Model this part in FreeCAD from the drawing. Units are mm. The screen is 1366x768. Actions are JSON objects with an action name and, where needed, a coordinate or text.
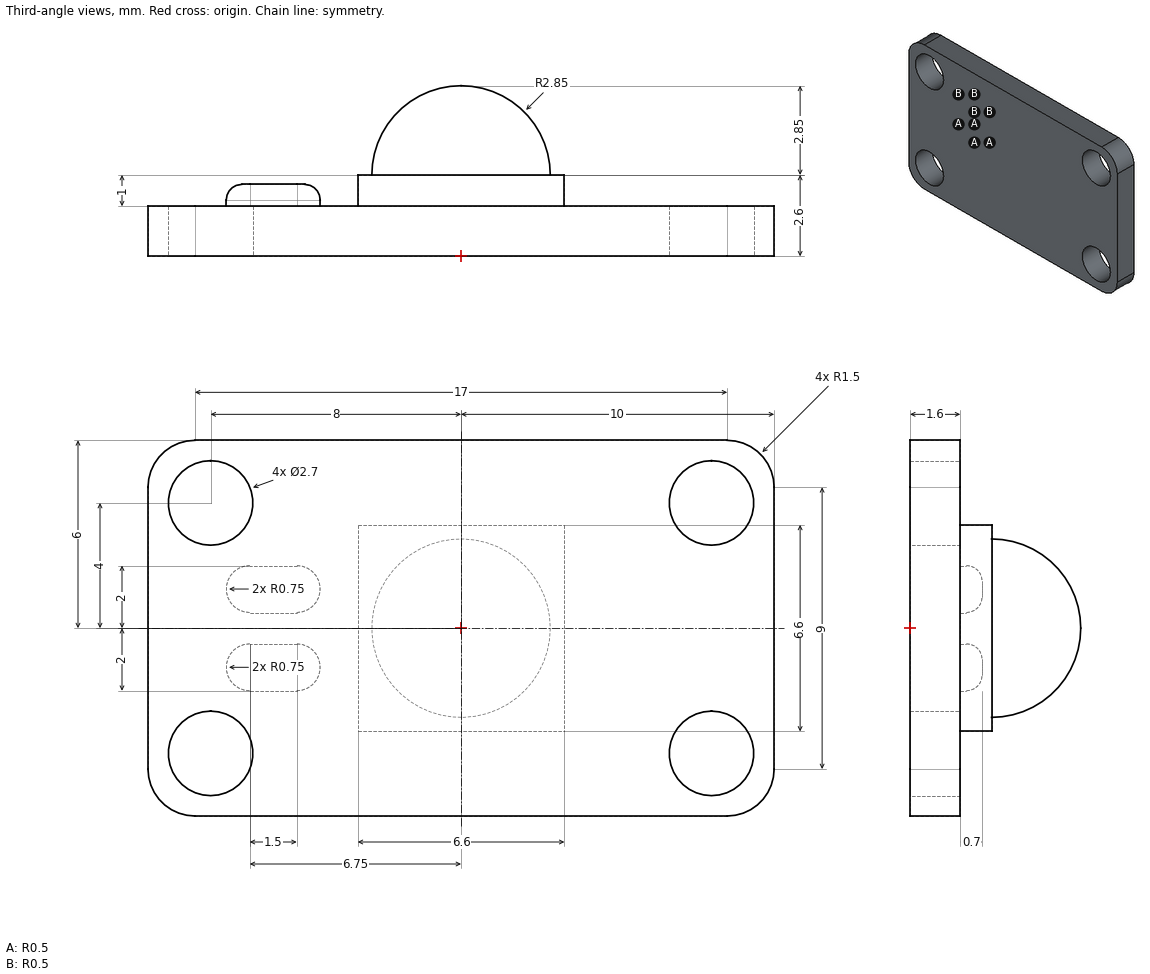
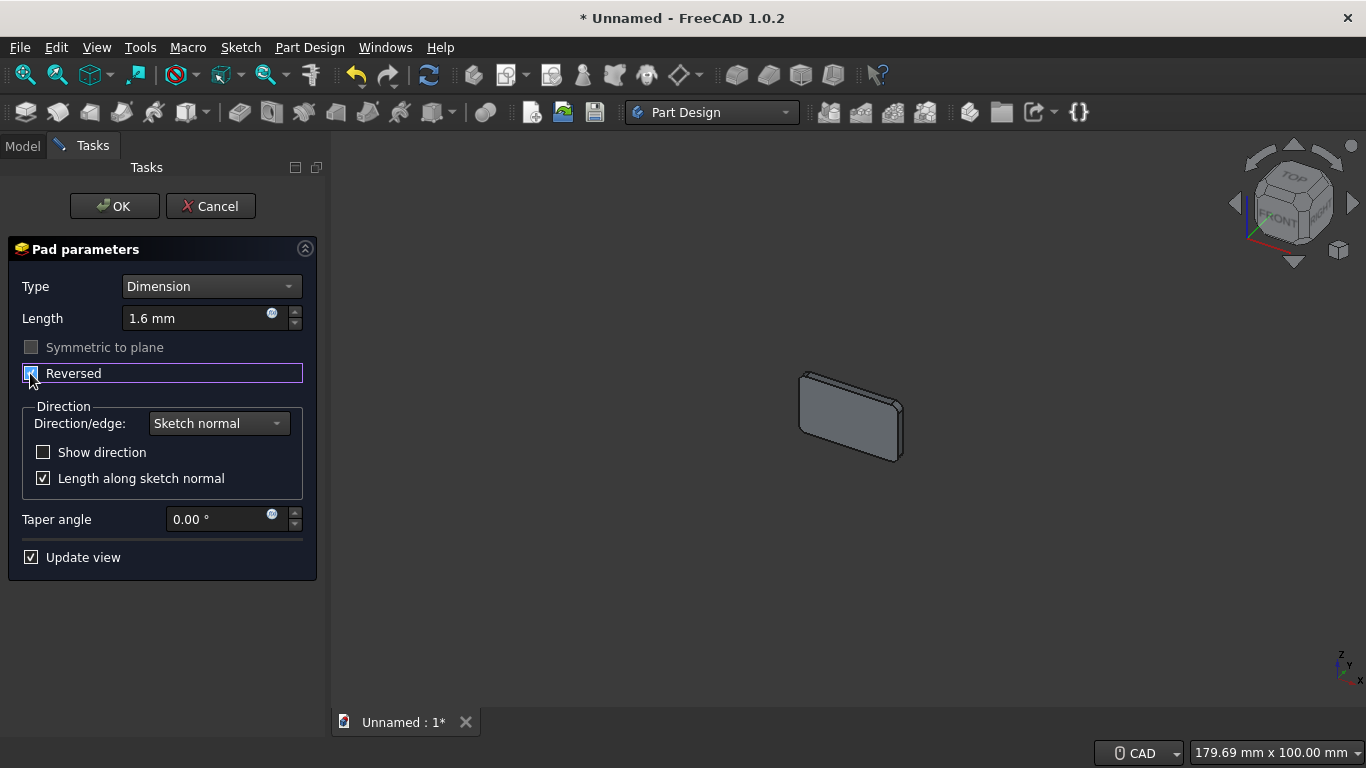
{"action": "left_click", "coordinate": [115, 206]}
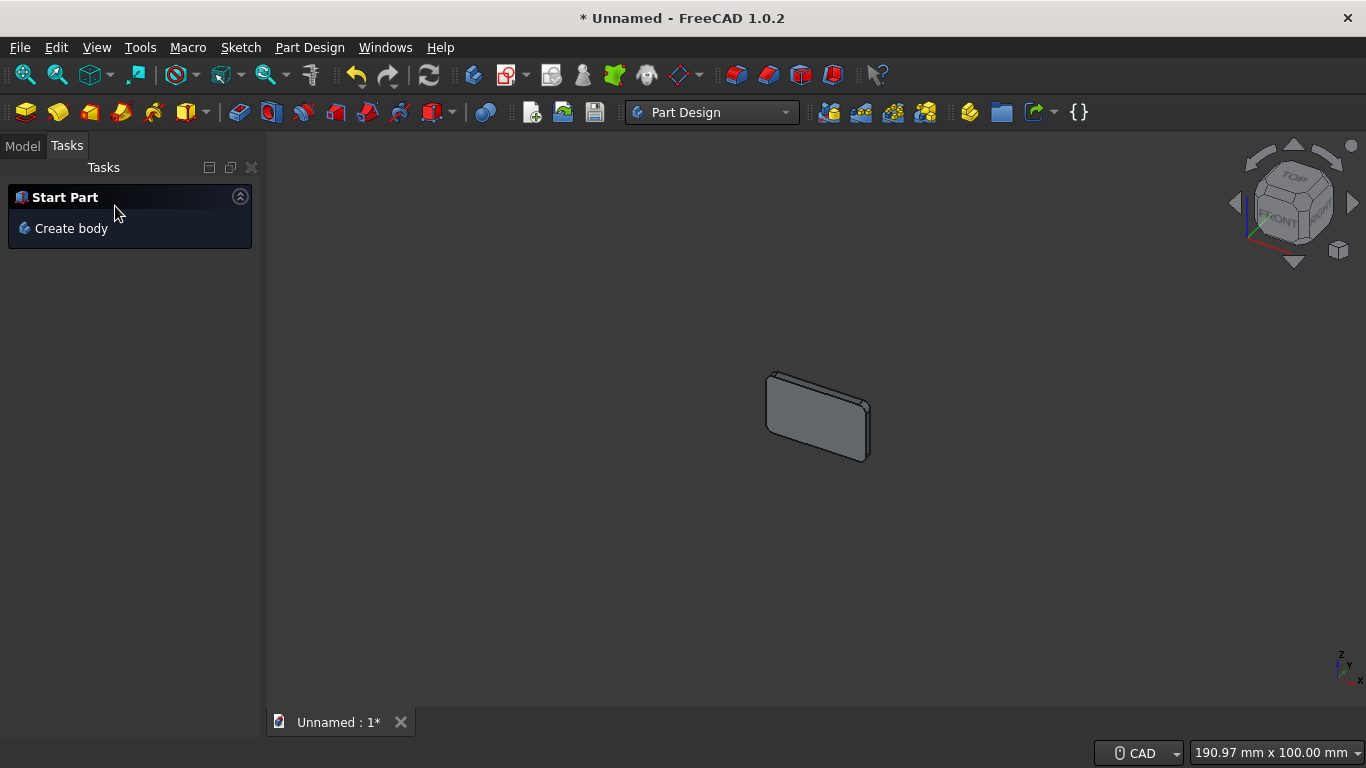
{"action": "key", "text": "v f"}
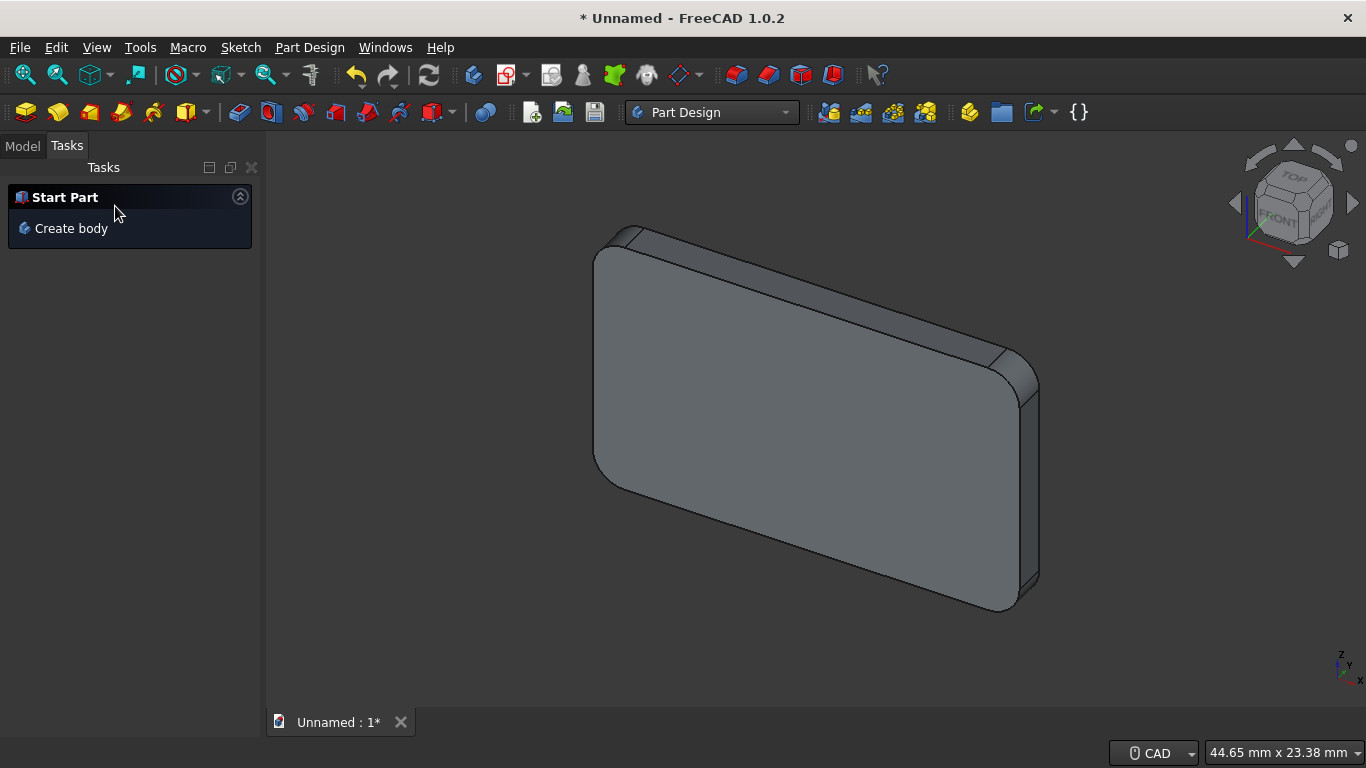
{"action": "left_click", "coordinate": [506, 76]}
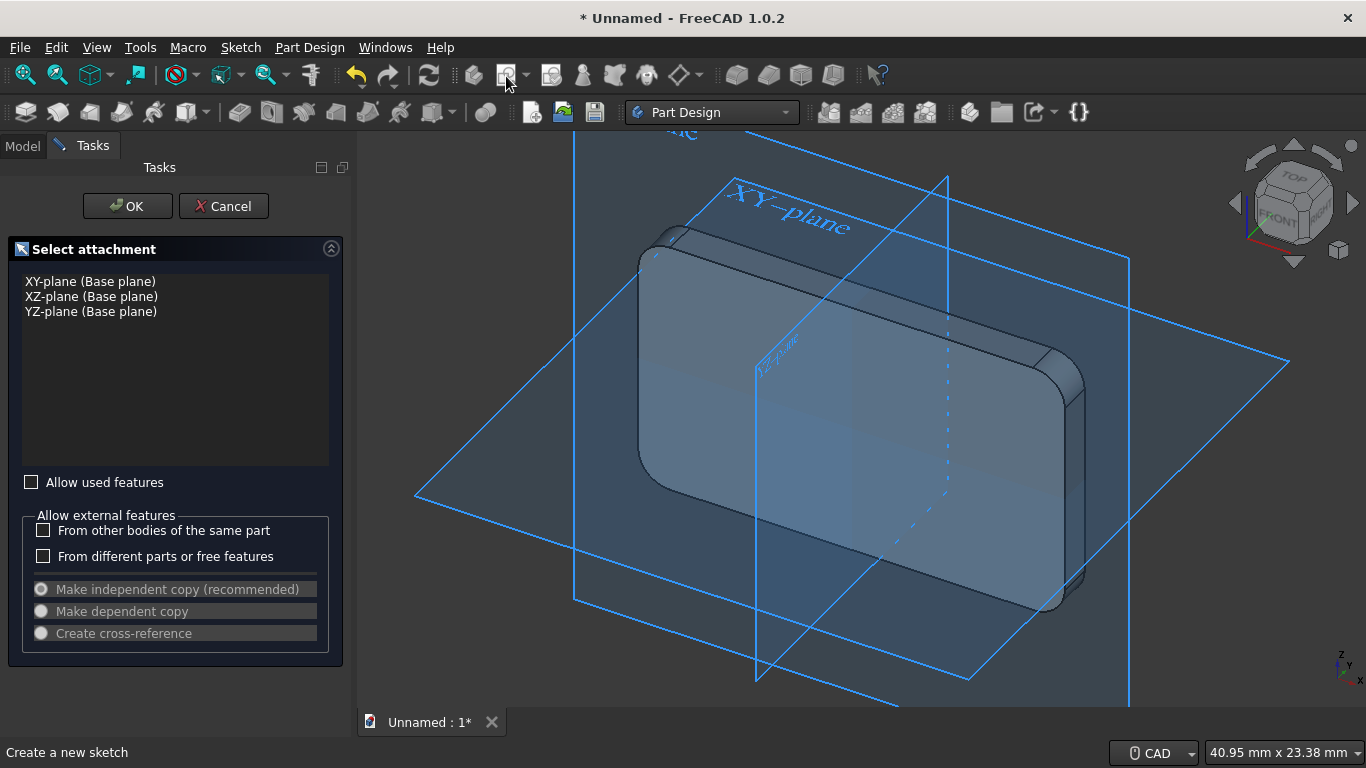
{"action": "left_click", "coordinate": [82, 296]}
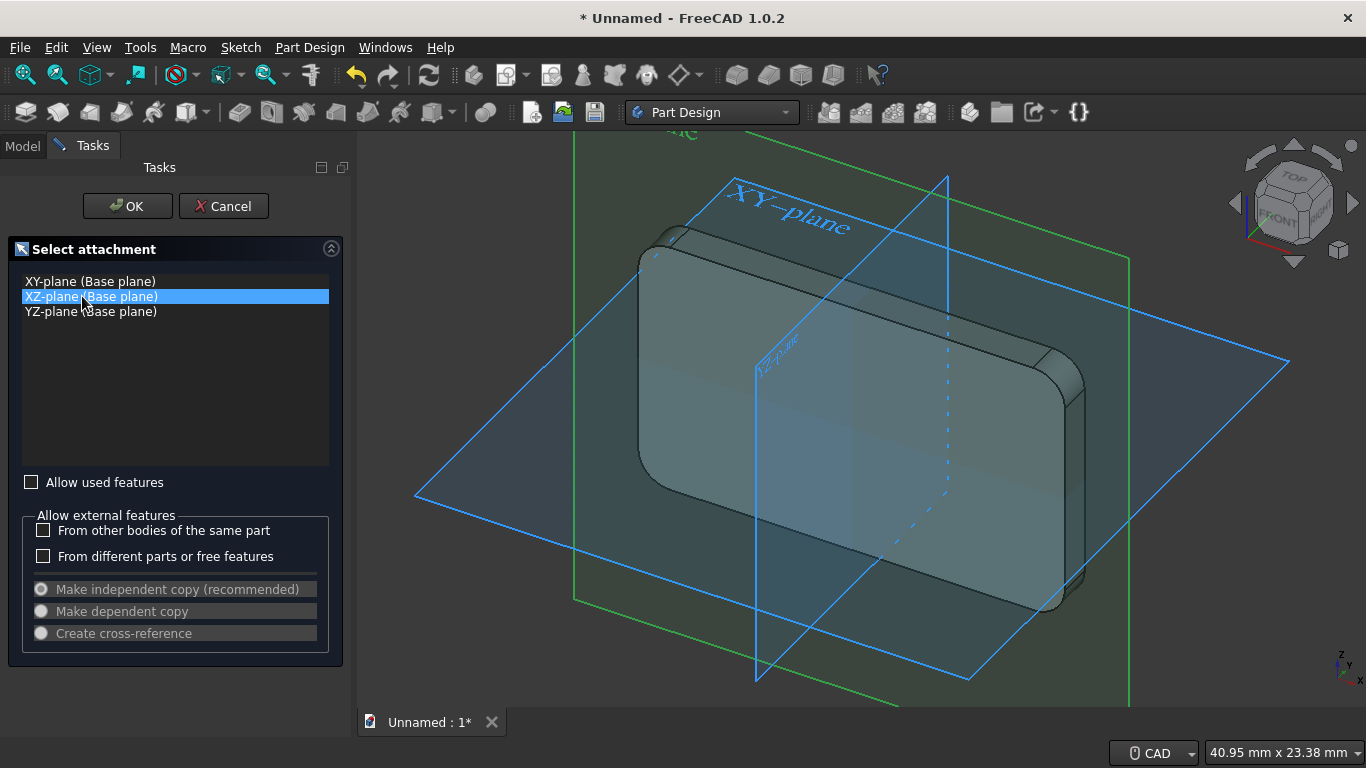
{"action": "left_click", "coordinate": [128, 206]}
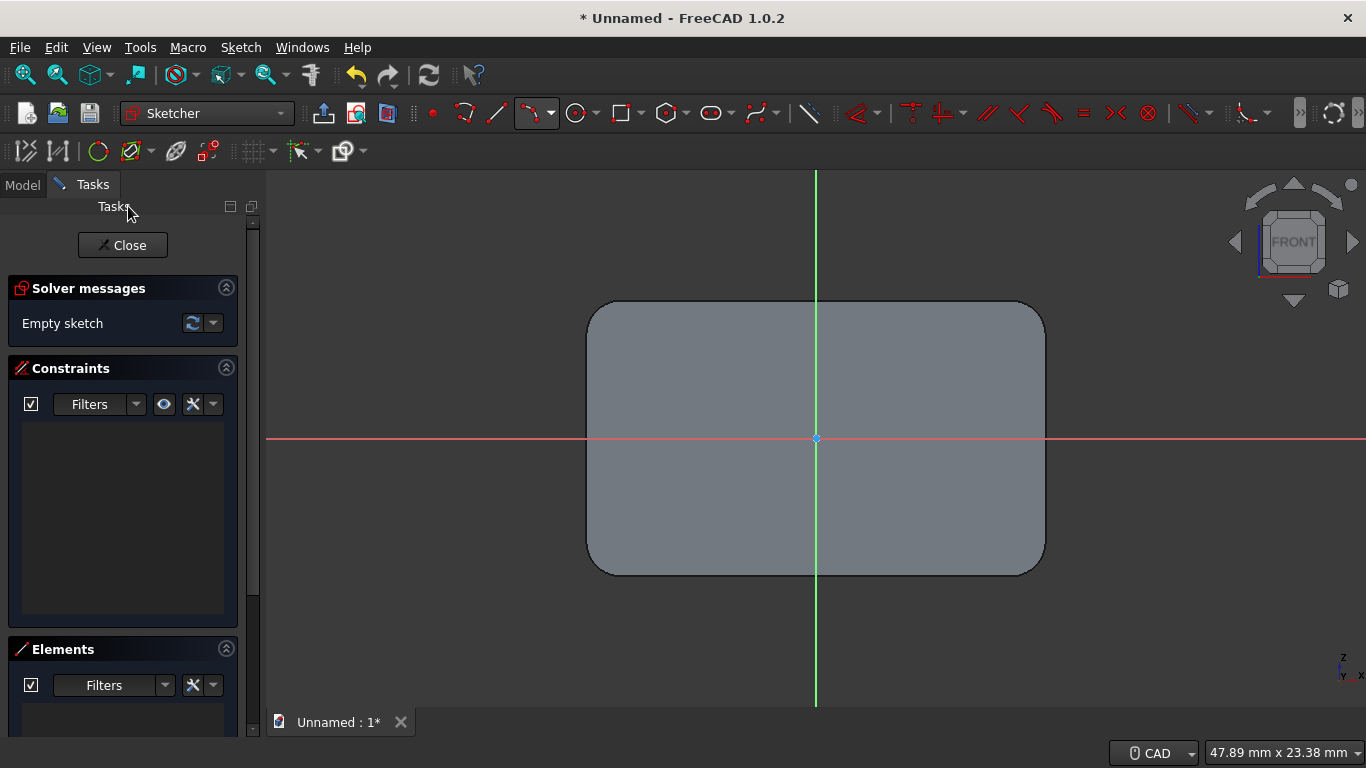
{"action": "scroll", "coordinate": [955, 439], "scroll_direction": "up", "scroll_amount": 2}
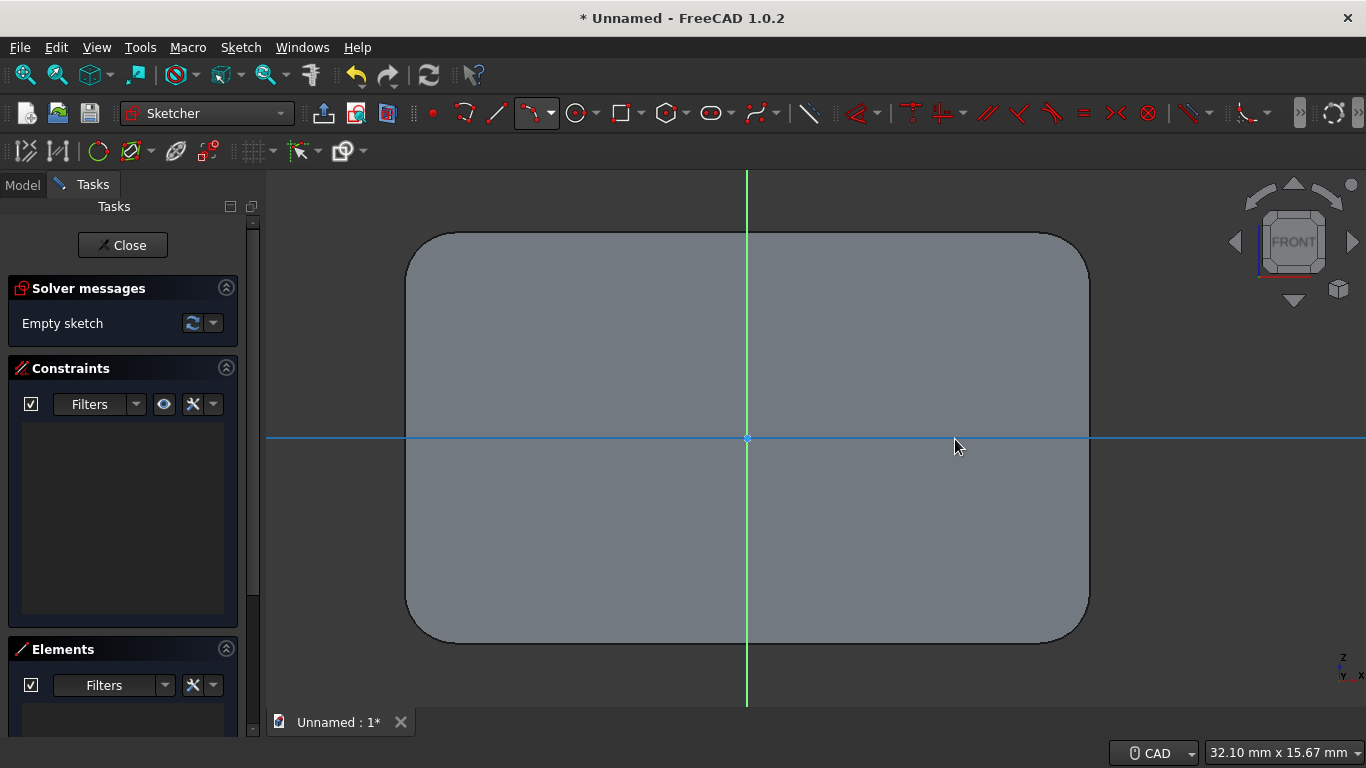
{"action": "left_click", "coordinate": [576, 114]}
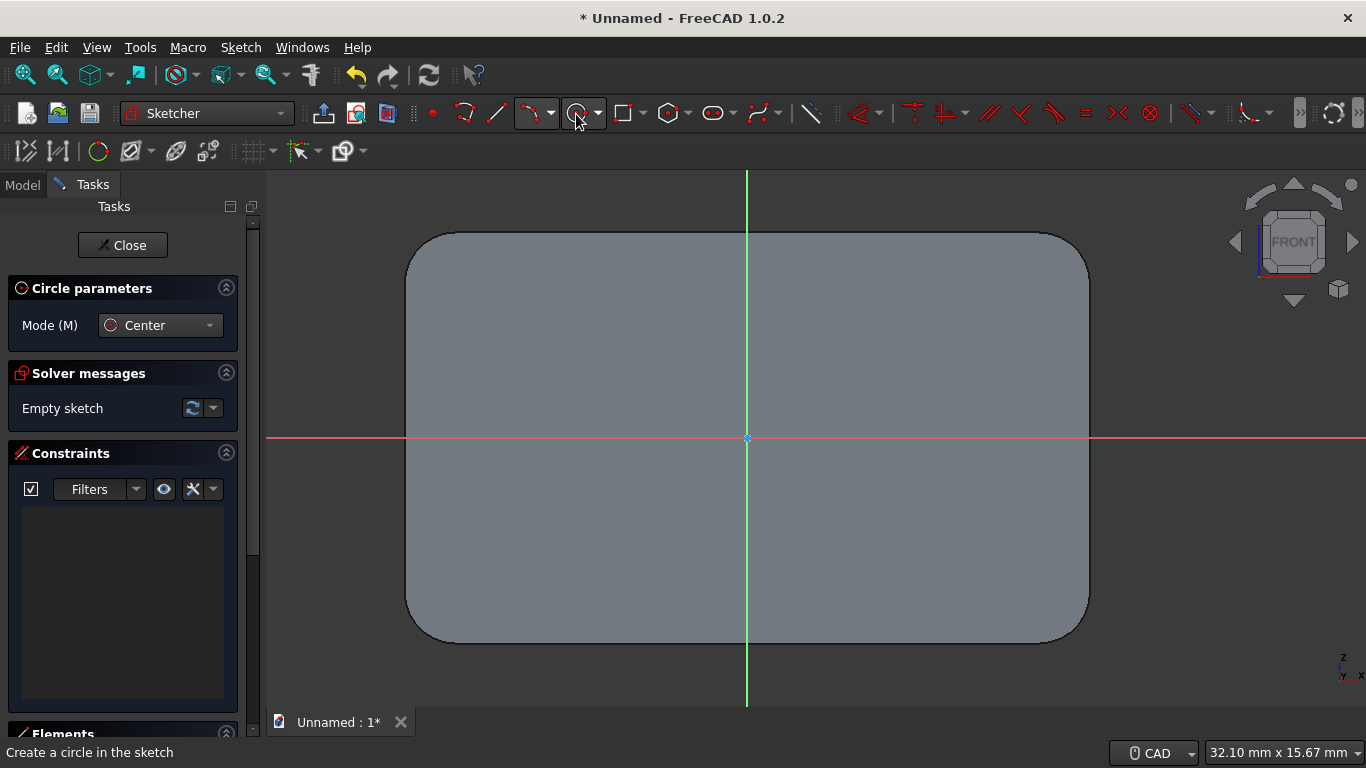
{"action": "left_click", "coordinate": [473, 301]}
{"action": "left_click", "coordinate": [506, 268]}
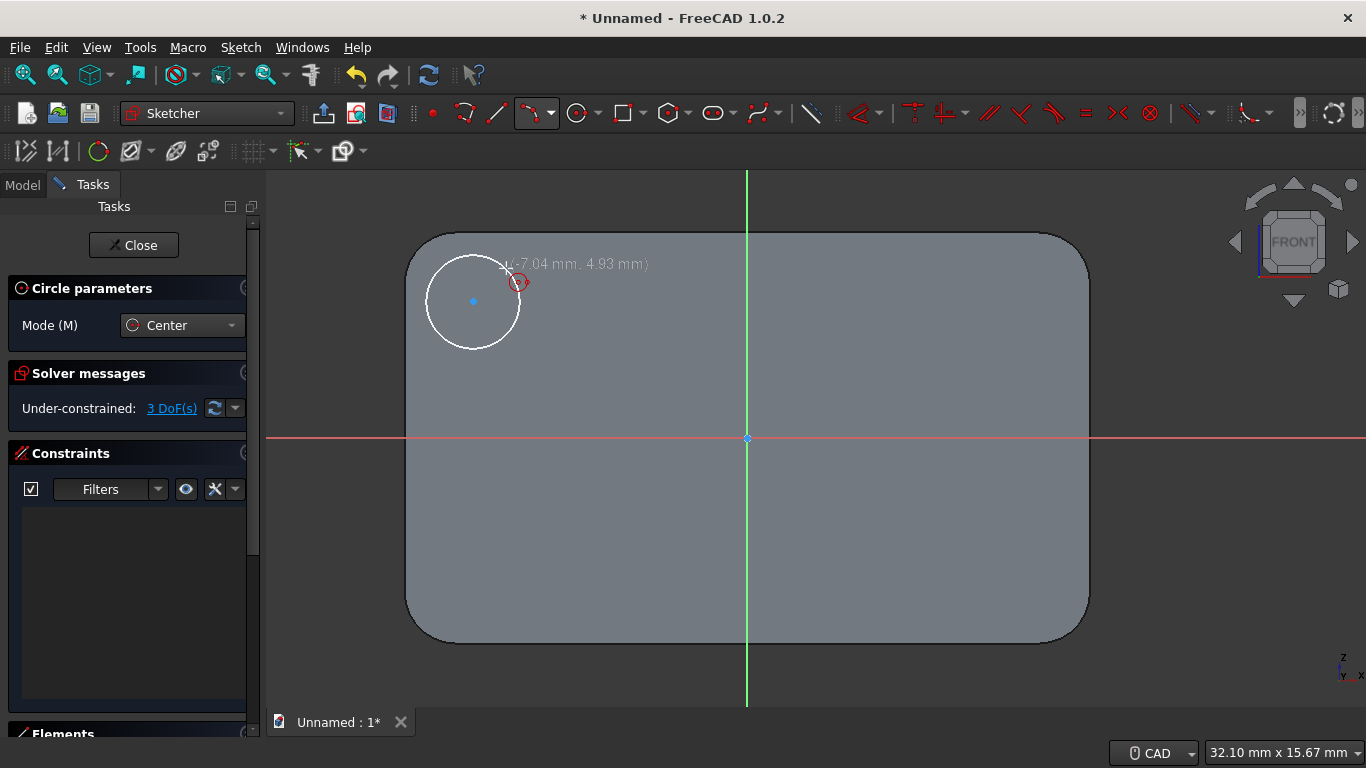
{"action": "left_click", "coordinate": [1021, 301]}
{"action": "left_click", "coordinate": [1054, 268]}